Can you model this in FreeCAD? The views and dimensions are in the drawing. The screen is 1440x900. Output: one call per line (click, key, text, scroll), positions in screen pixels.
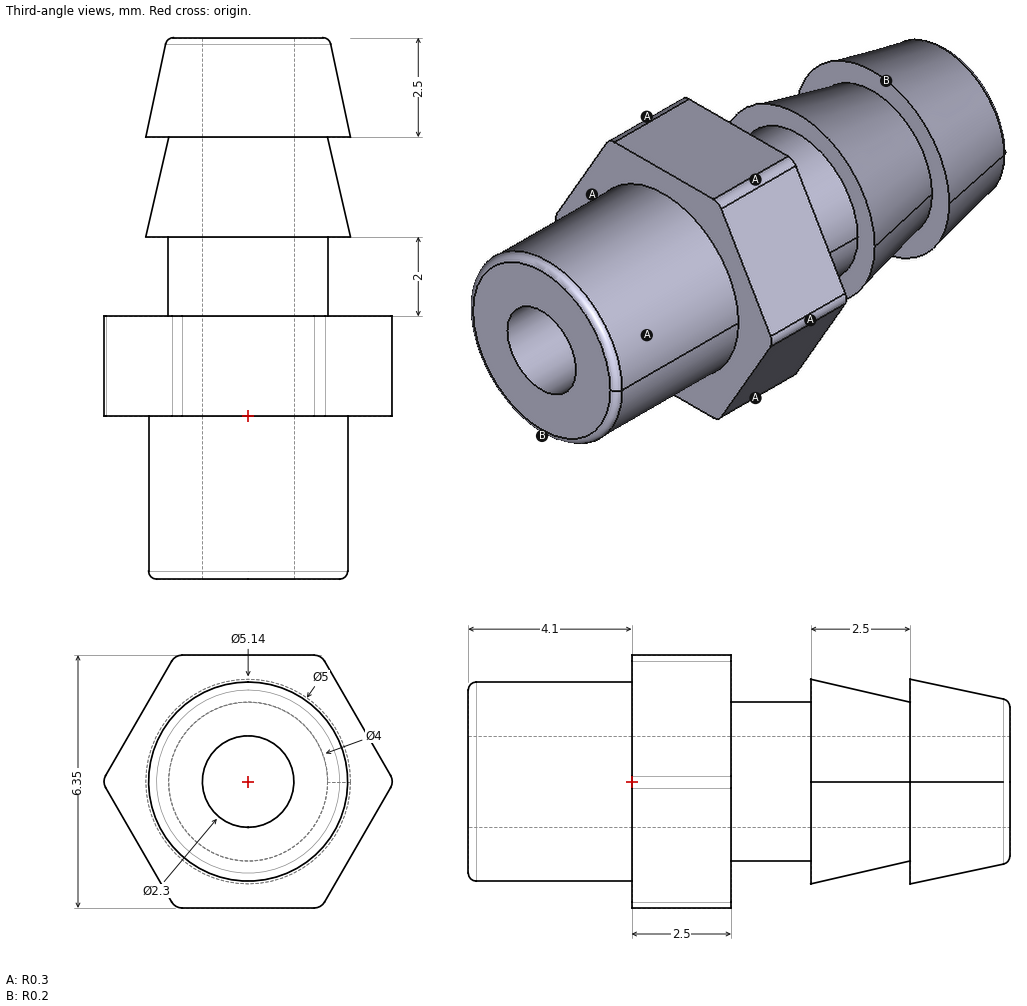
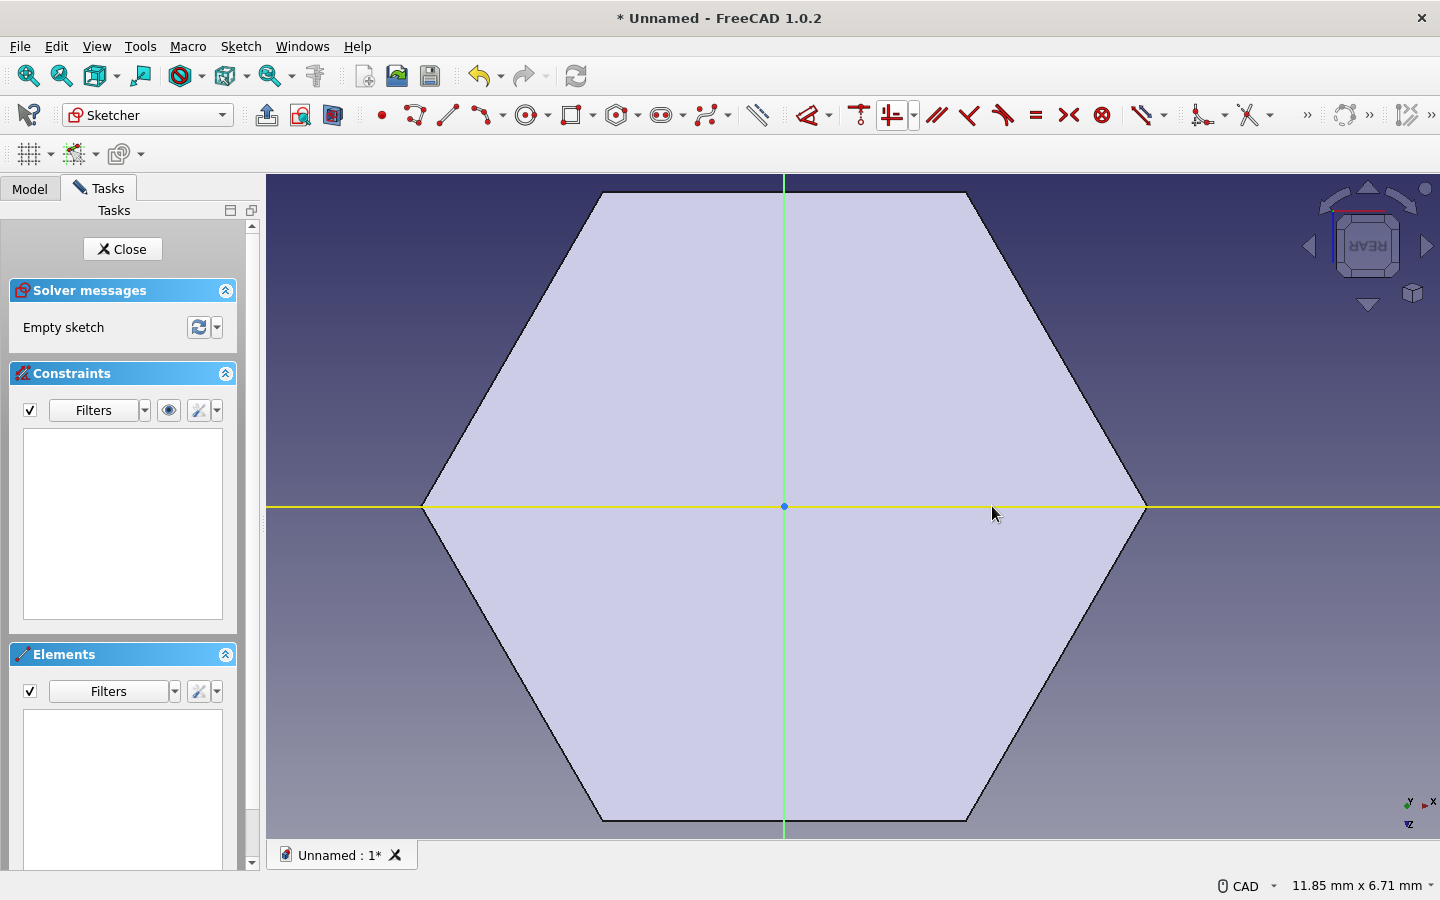
click(526, 116)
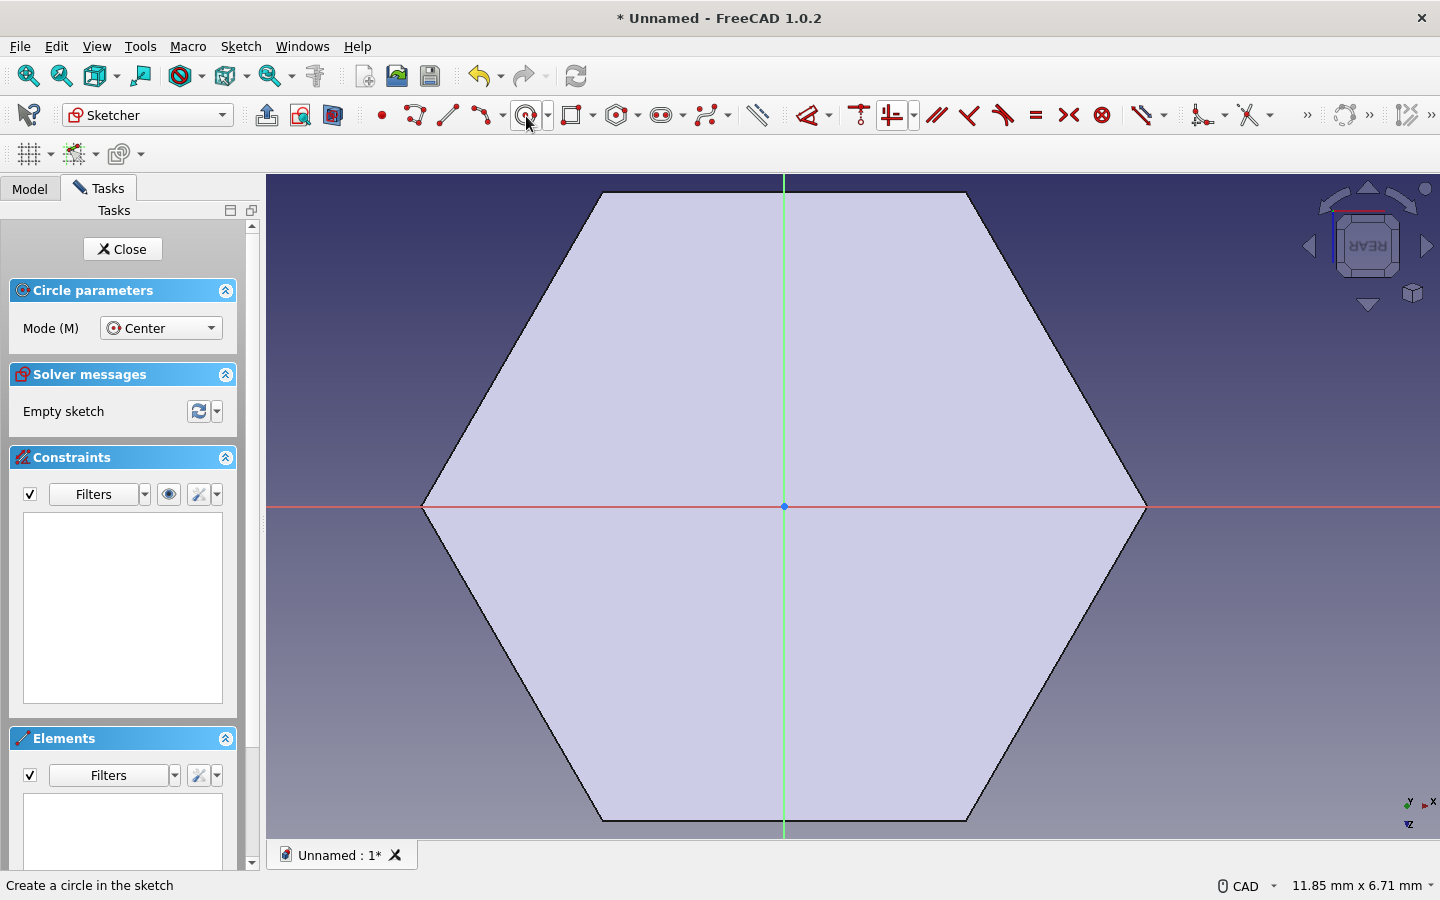
click(784, 506)
click(924, 366)
key(Escape)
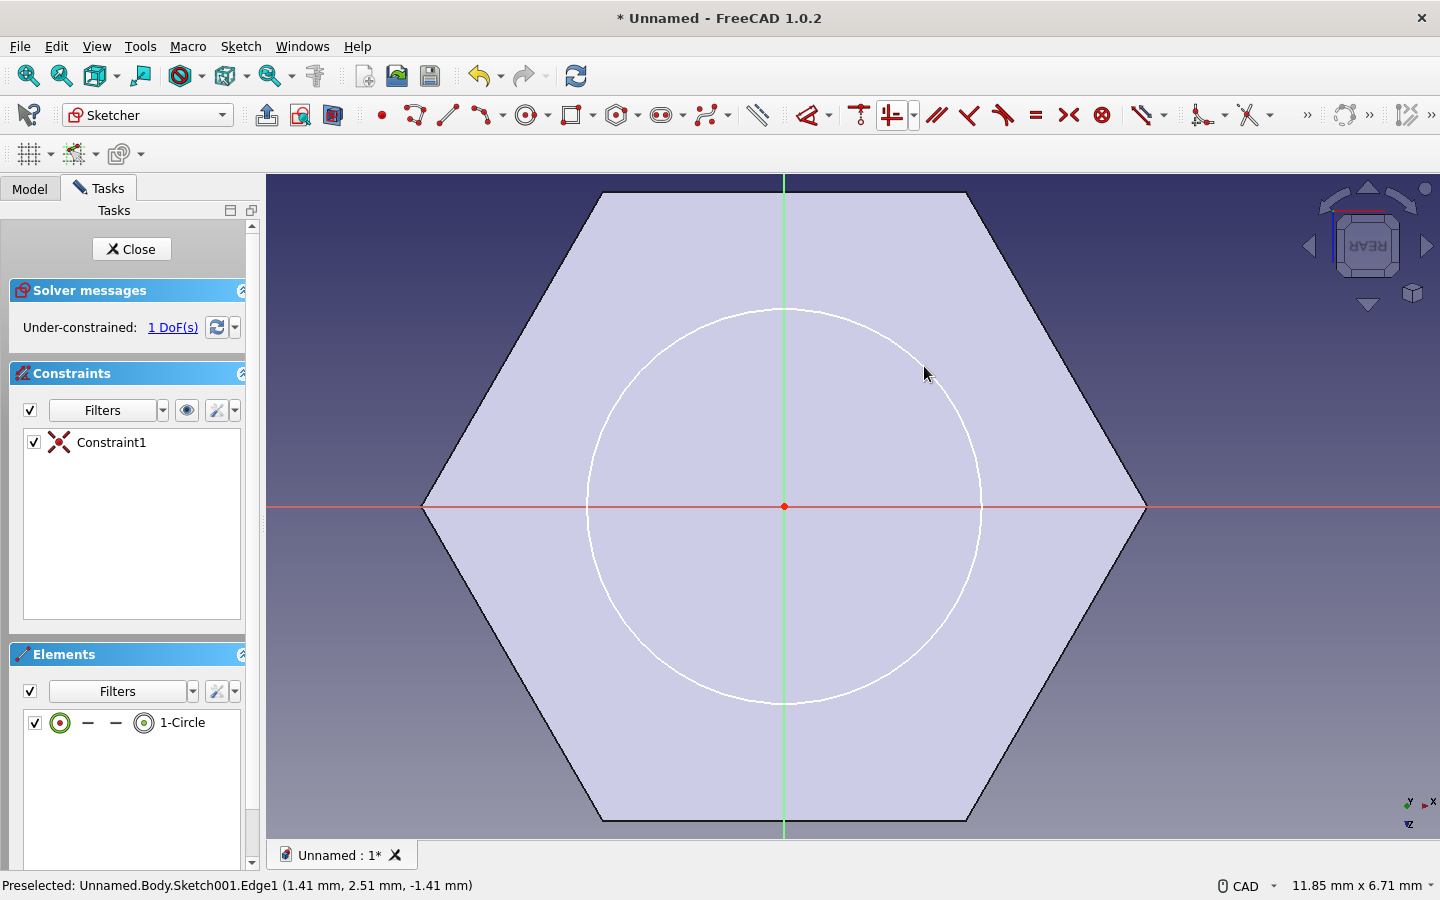
key(d)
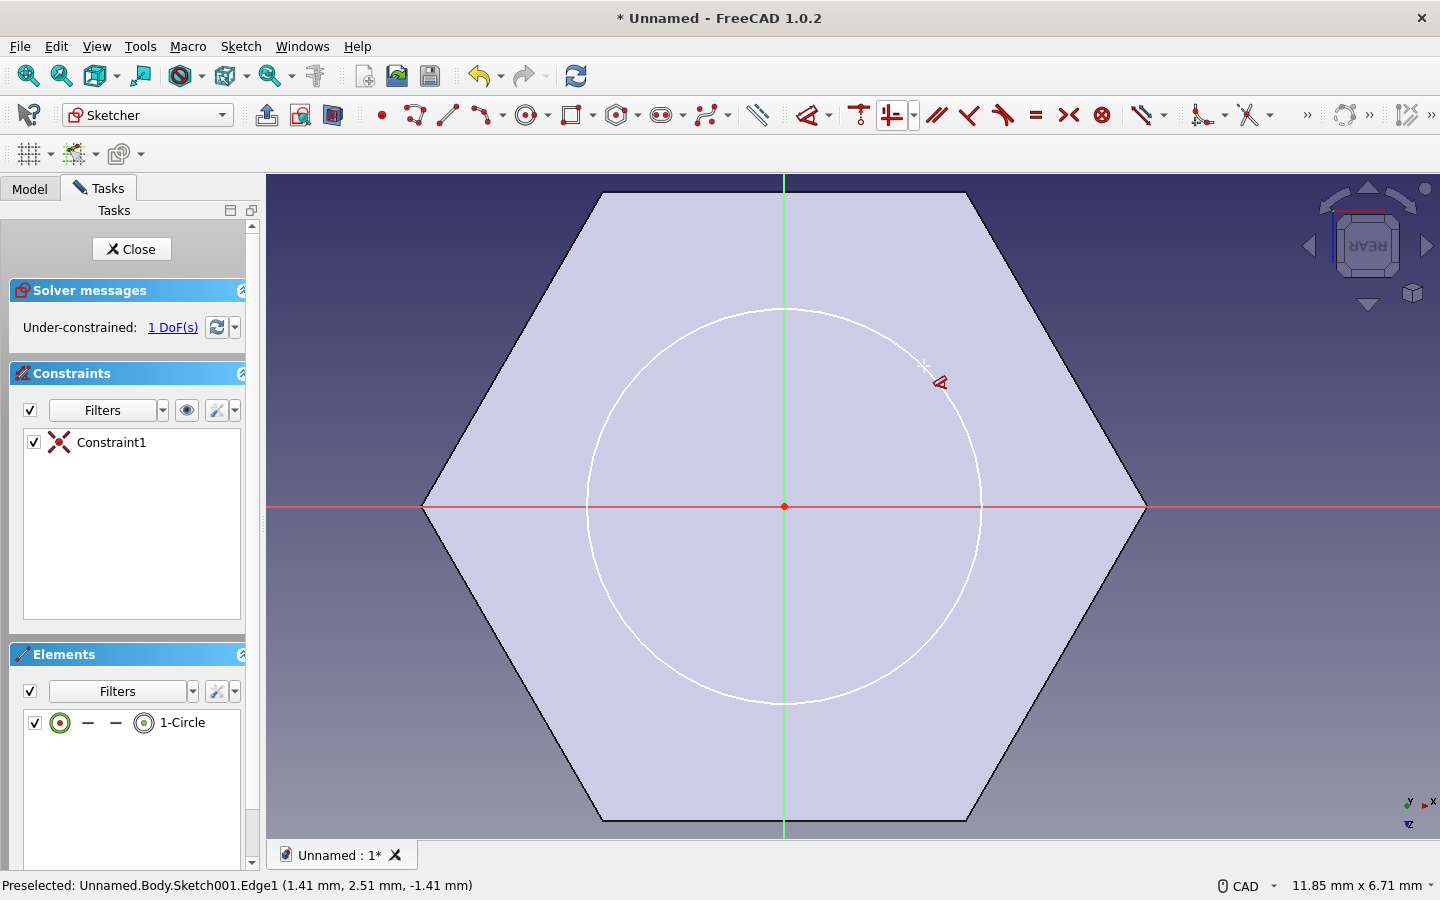
click(923, 366)
click(945, 343)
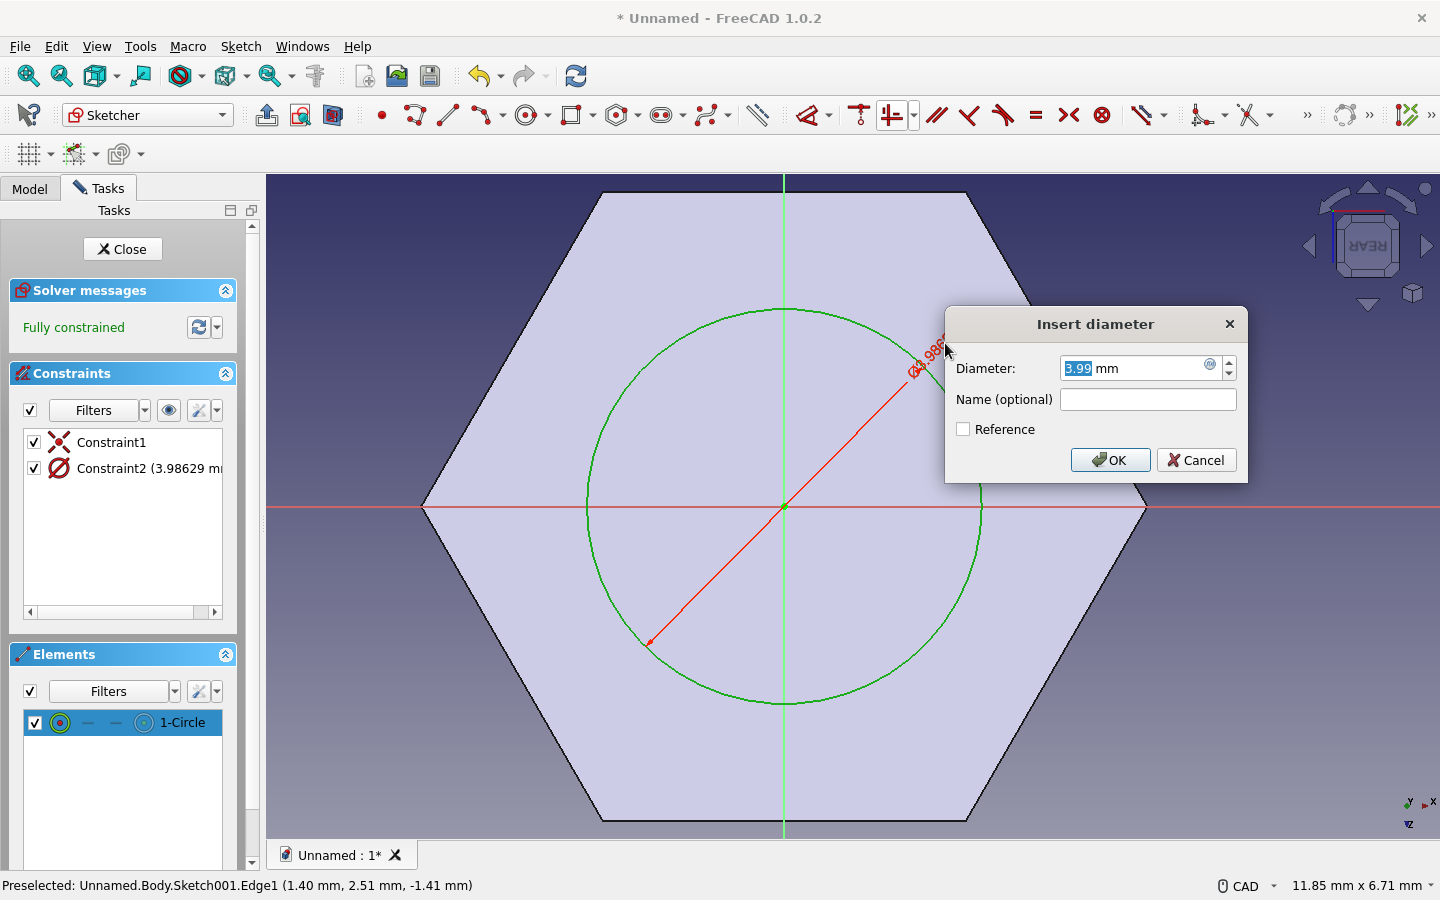
text(4)
key(Return)
key(Escape)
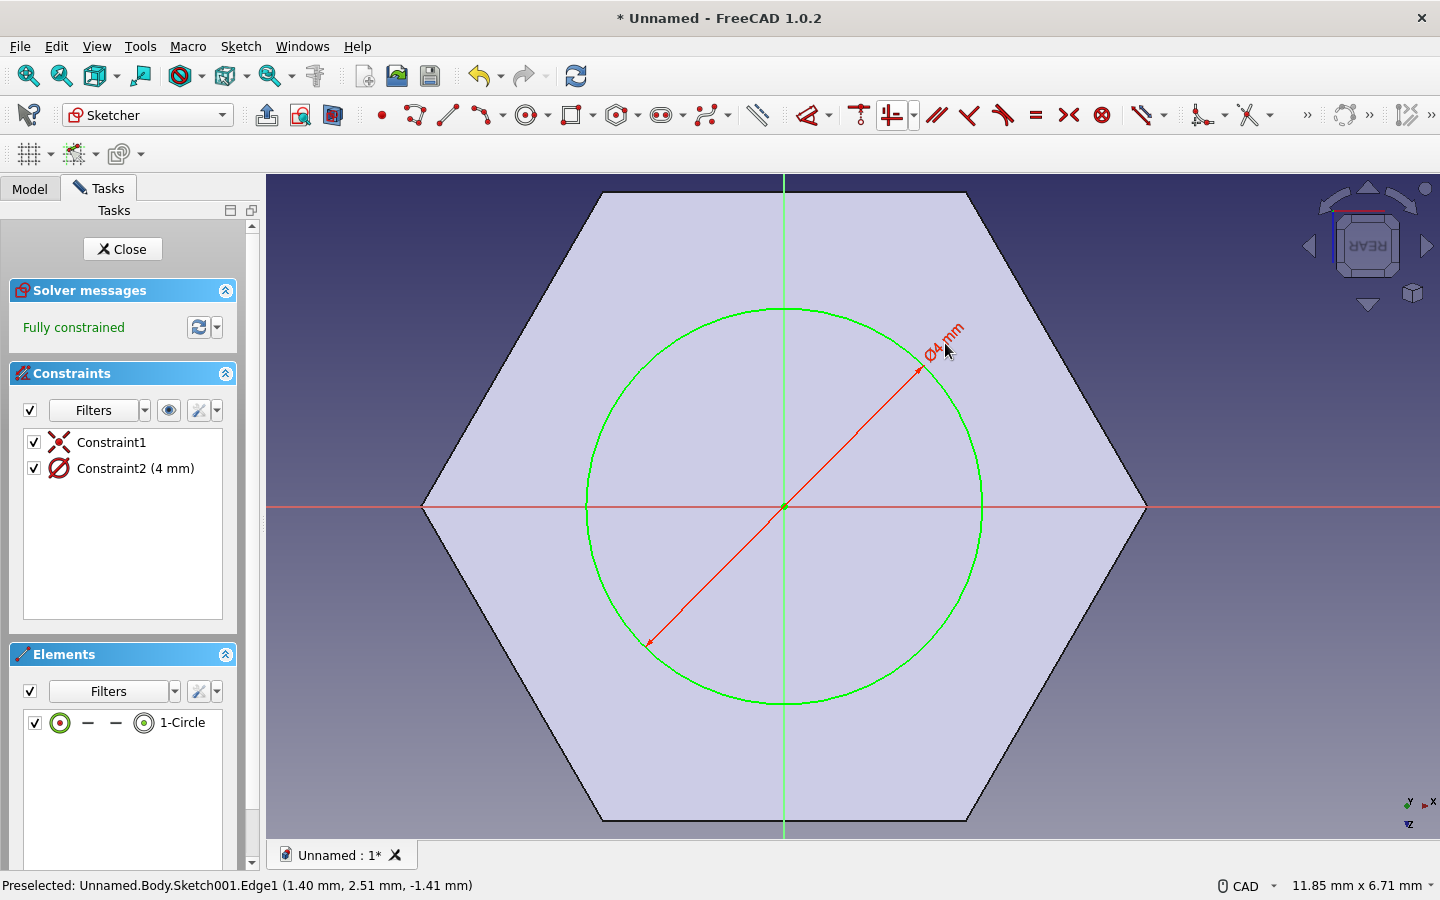
click(123, 249)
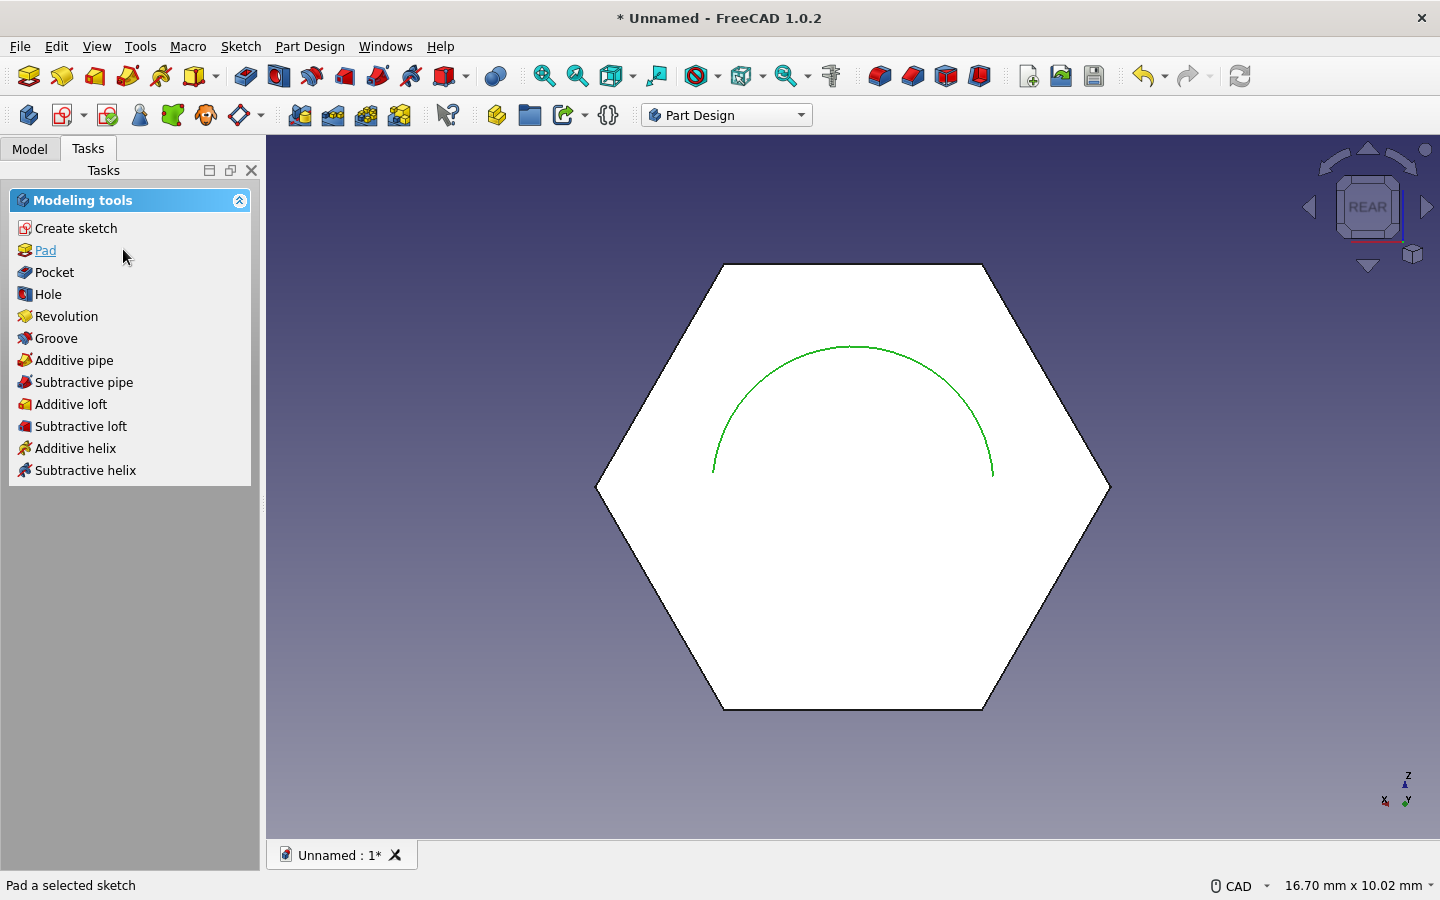
click(29, 76)